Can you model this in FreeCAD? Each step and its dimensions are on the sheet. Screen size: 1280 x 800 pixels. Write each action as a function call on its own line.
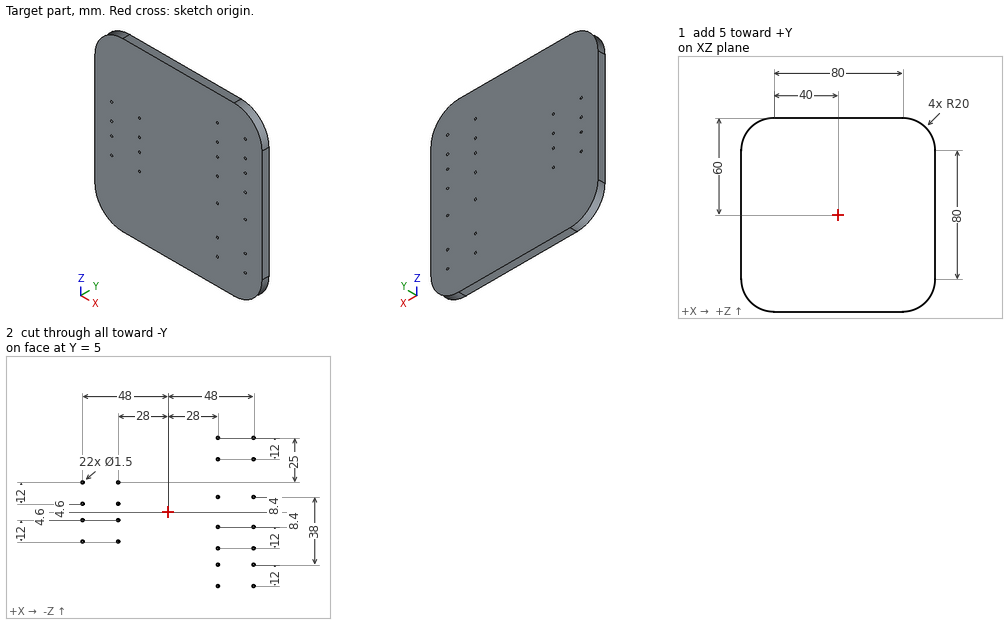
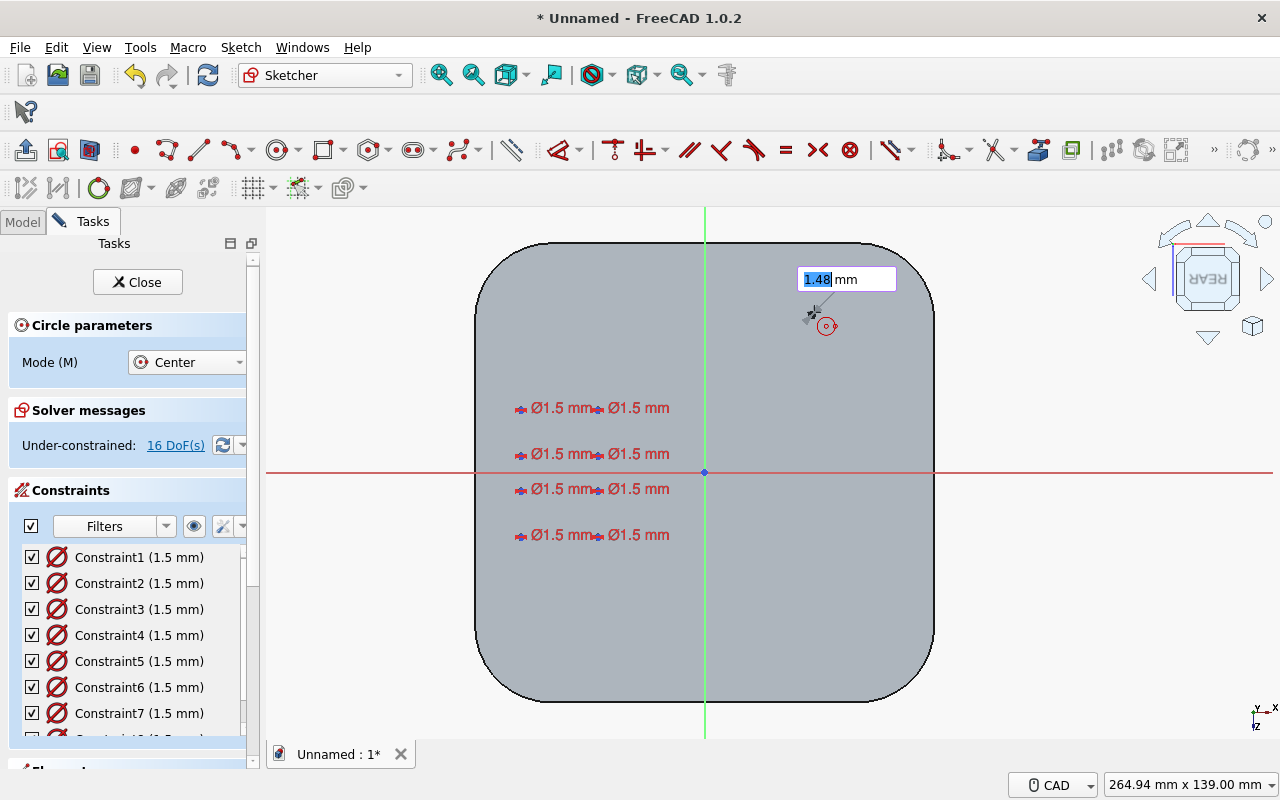
text(1.5)
key(Return)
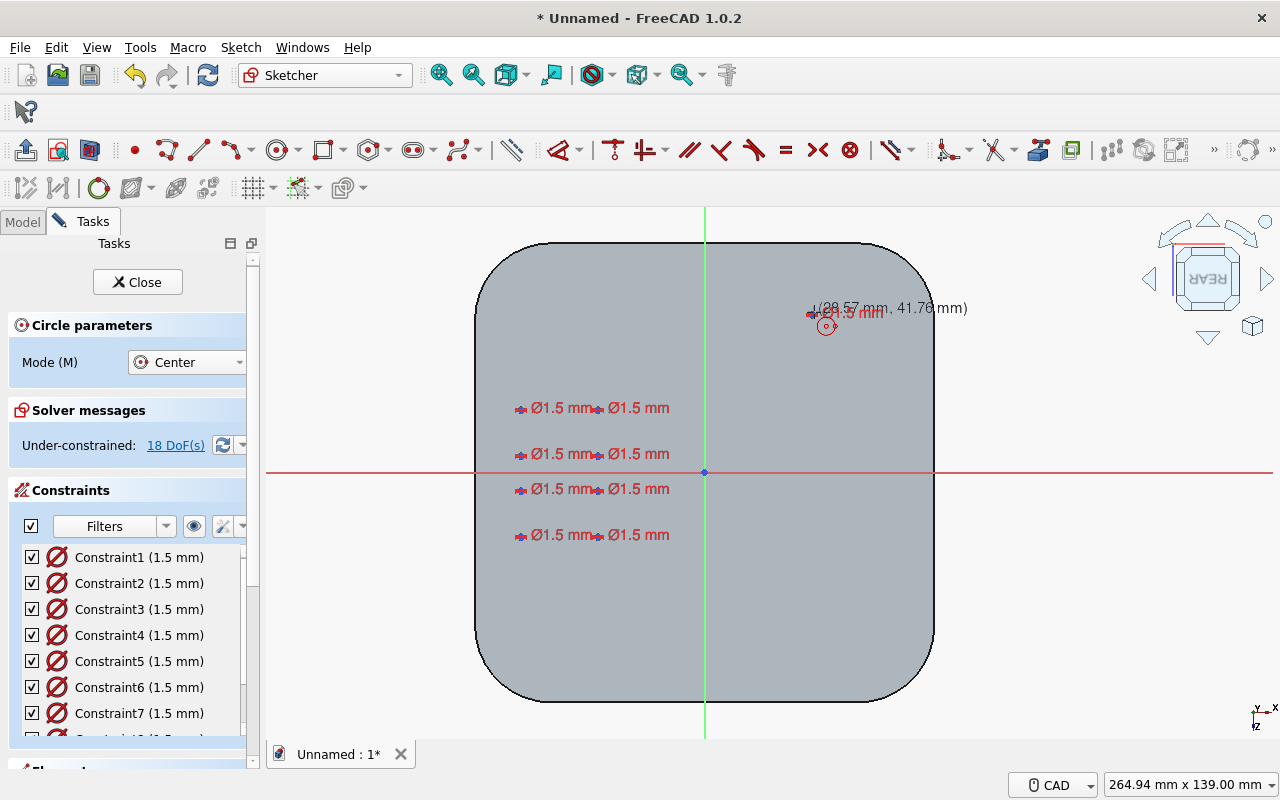
scroll(888, 314, up, 11)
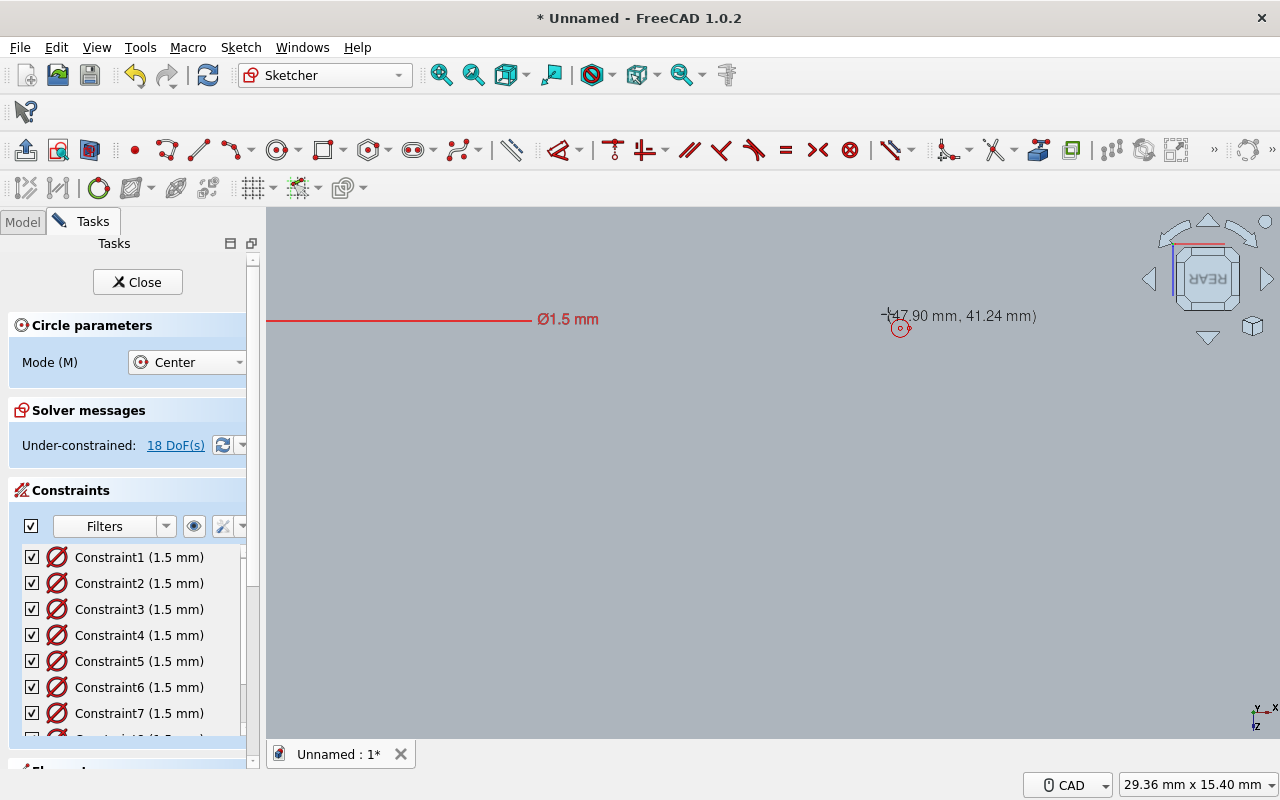
scroll(888, 314, down, 11)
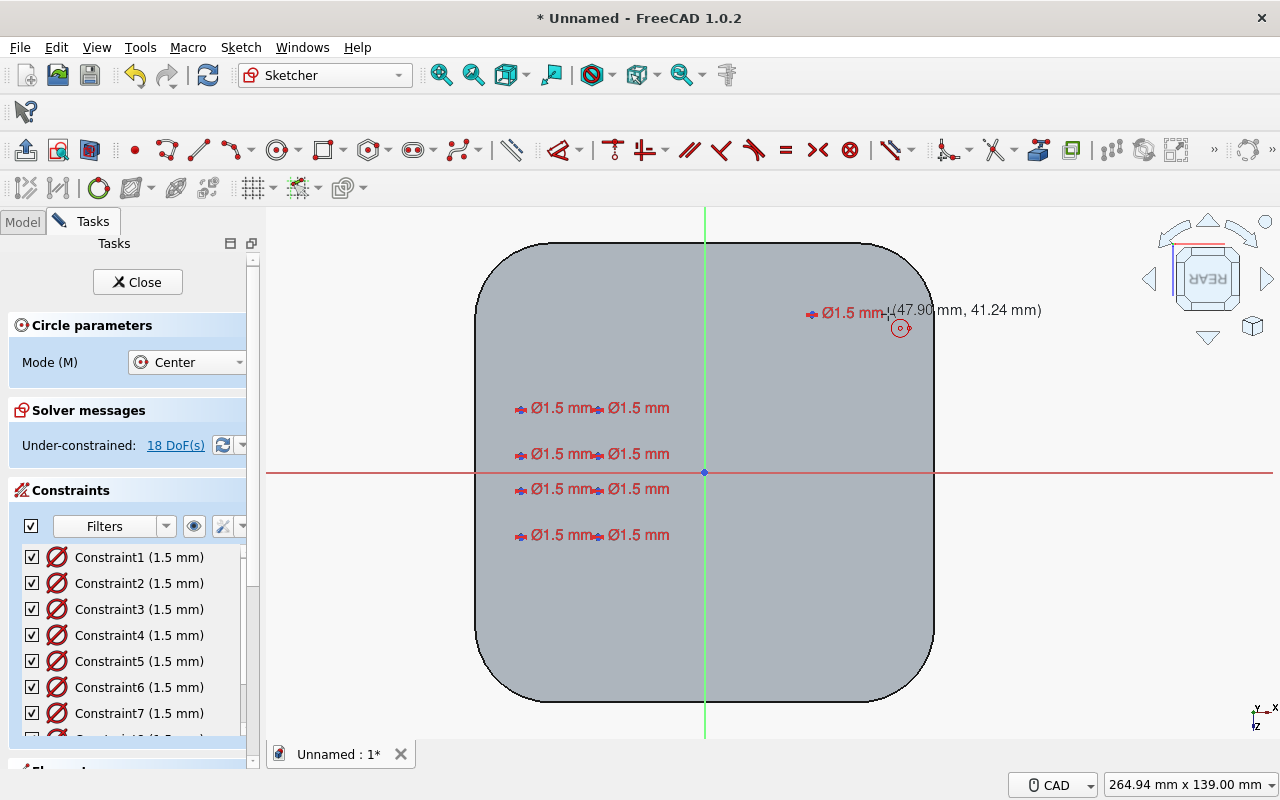
click(888, 314)
move(890, 312)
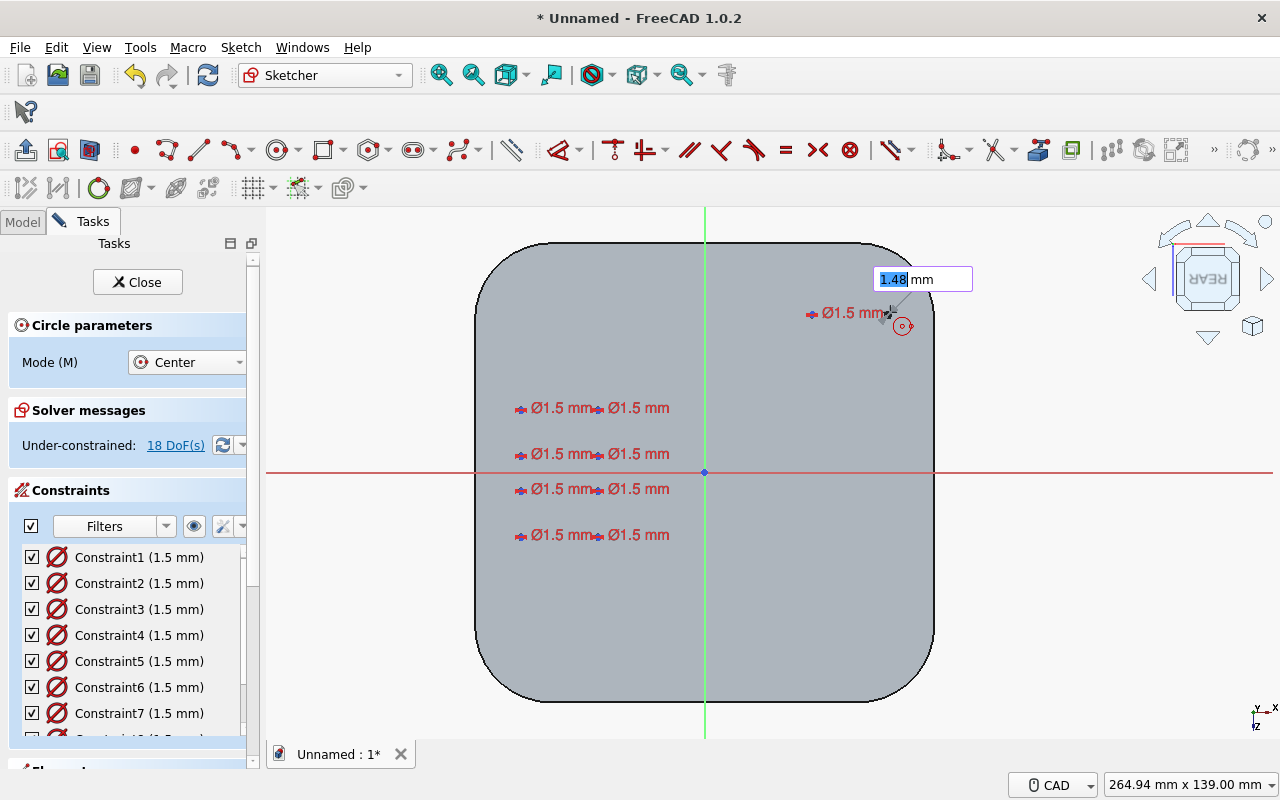
text(1.5)
key(Return)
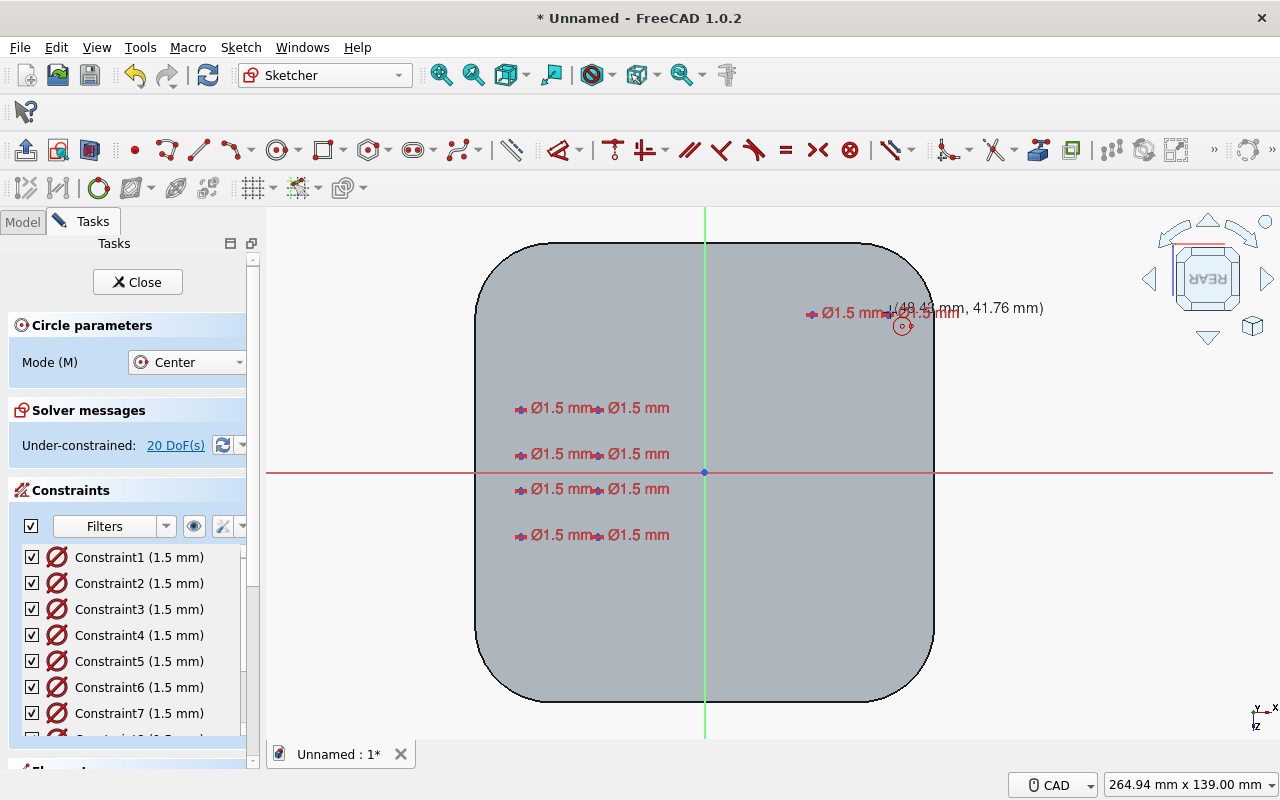
scroll(812, 360, up, 11)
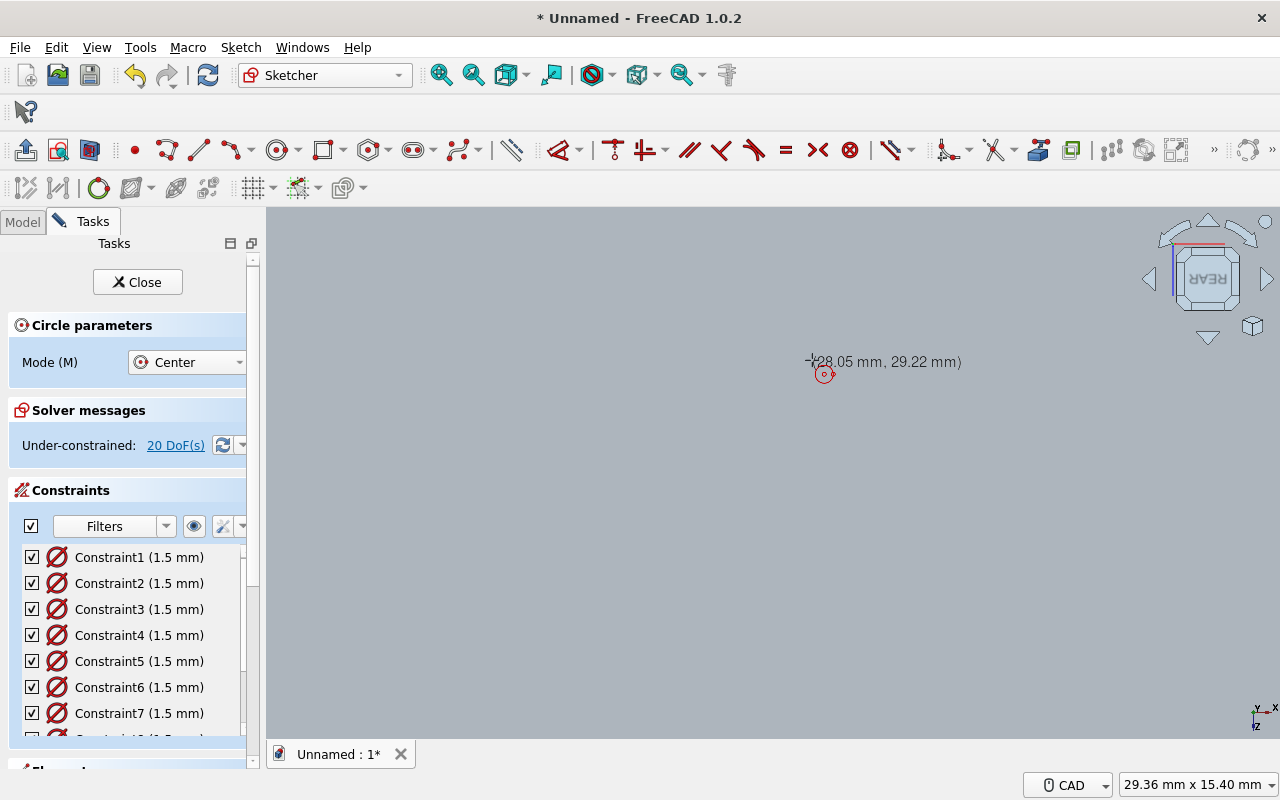
scroll(812, 360, down, 11)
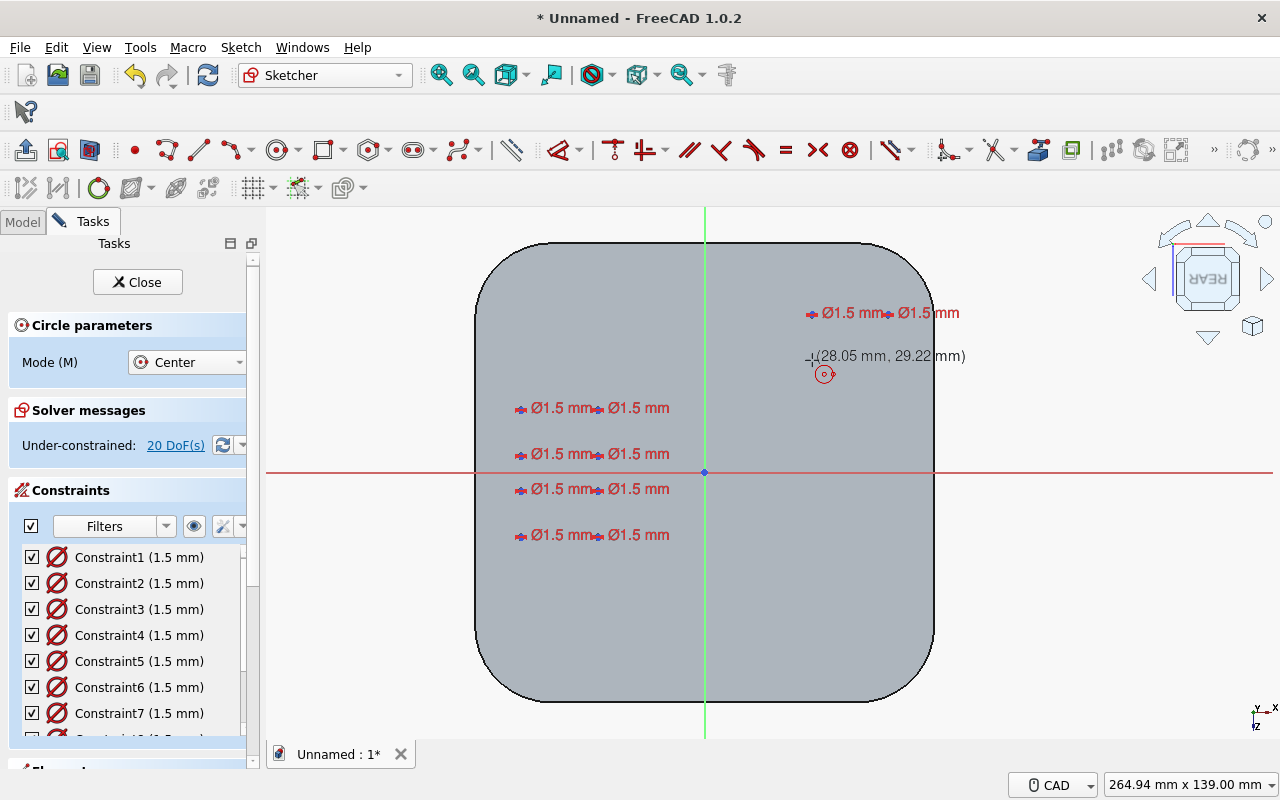
click(812, 360)
move(814, 358)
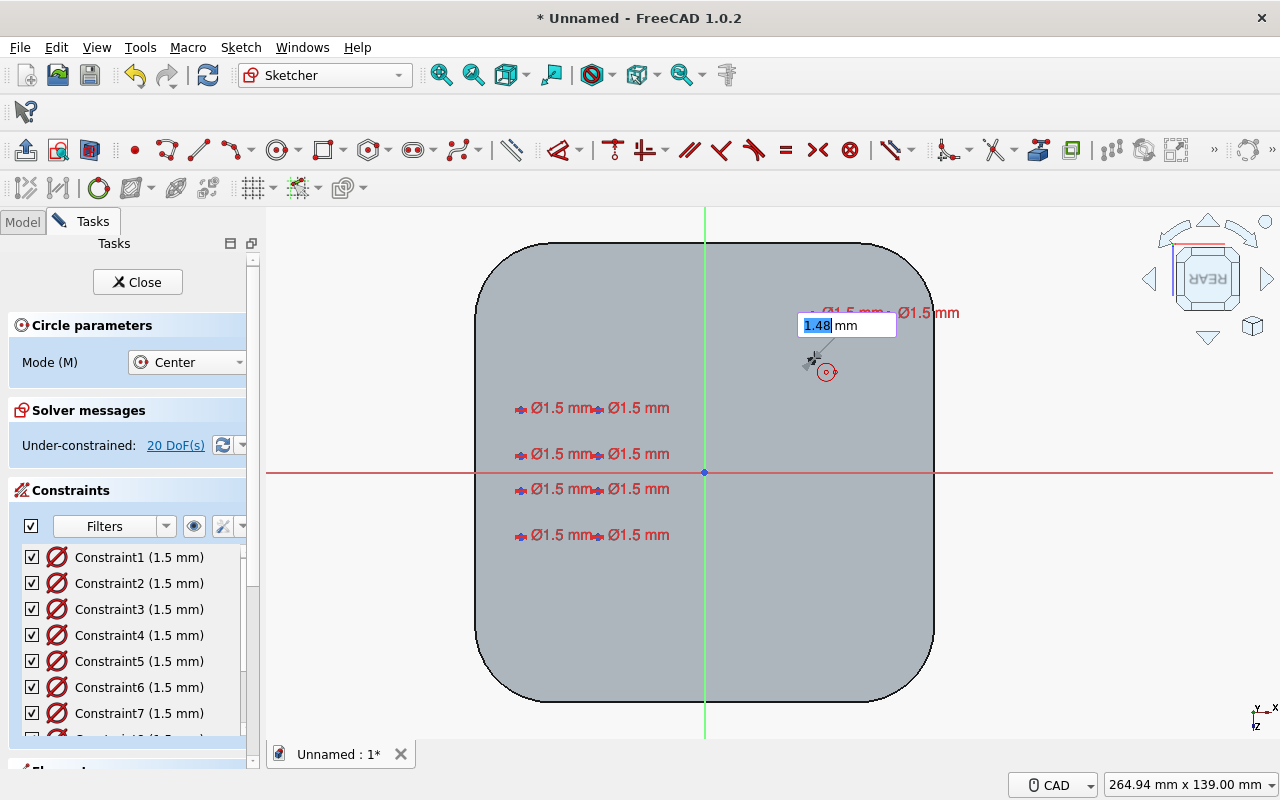
text(1.5)
key(Return)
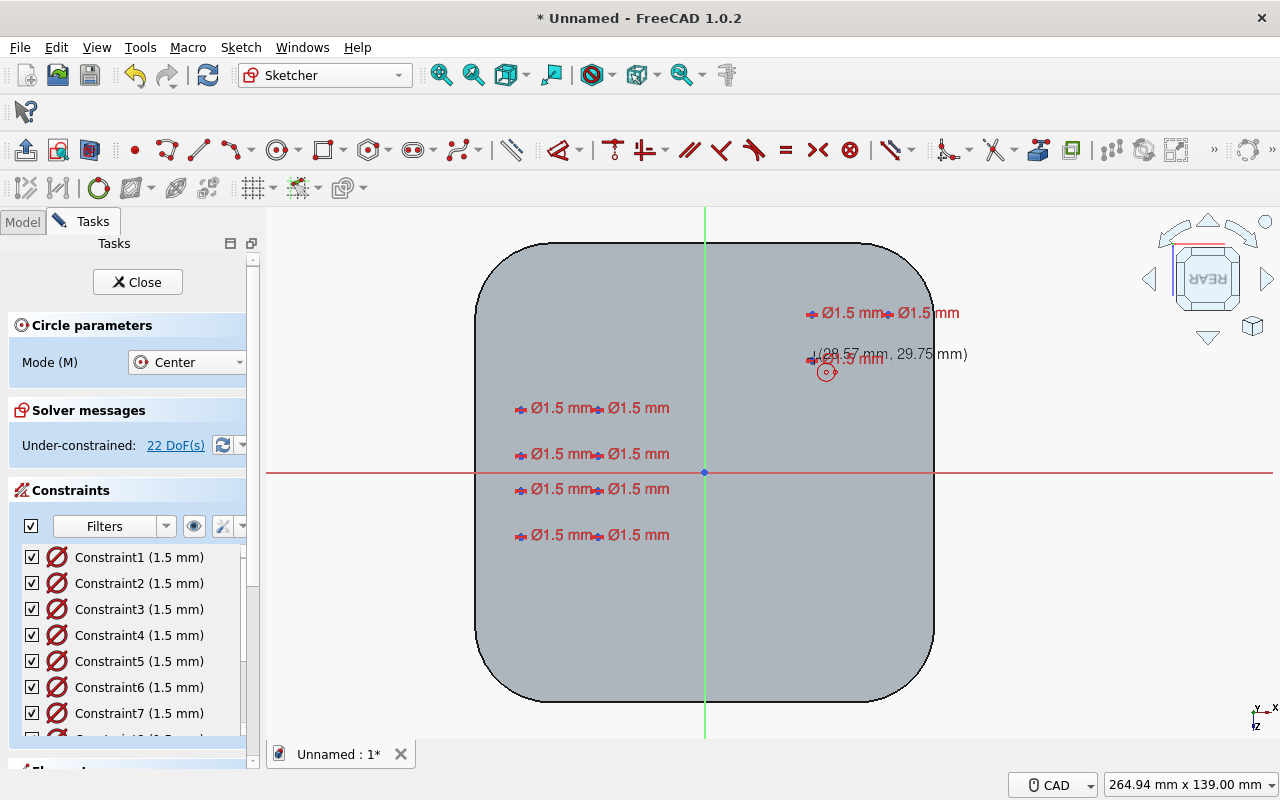
scroll(888, 360, up, 11)